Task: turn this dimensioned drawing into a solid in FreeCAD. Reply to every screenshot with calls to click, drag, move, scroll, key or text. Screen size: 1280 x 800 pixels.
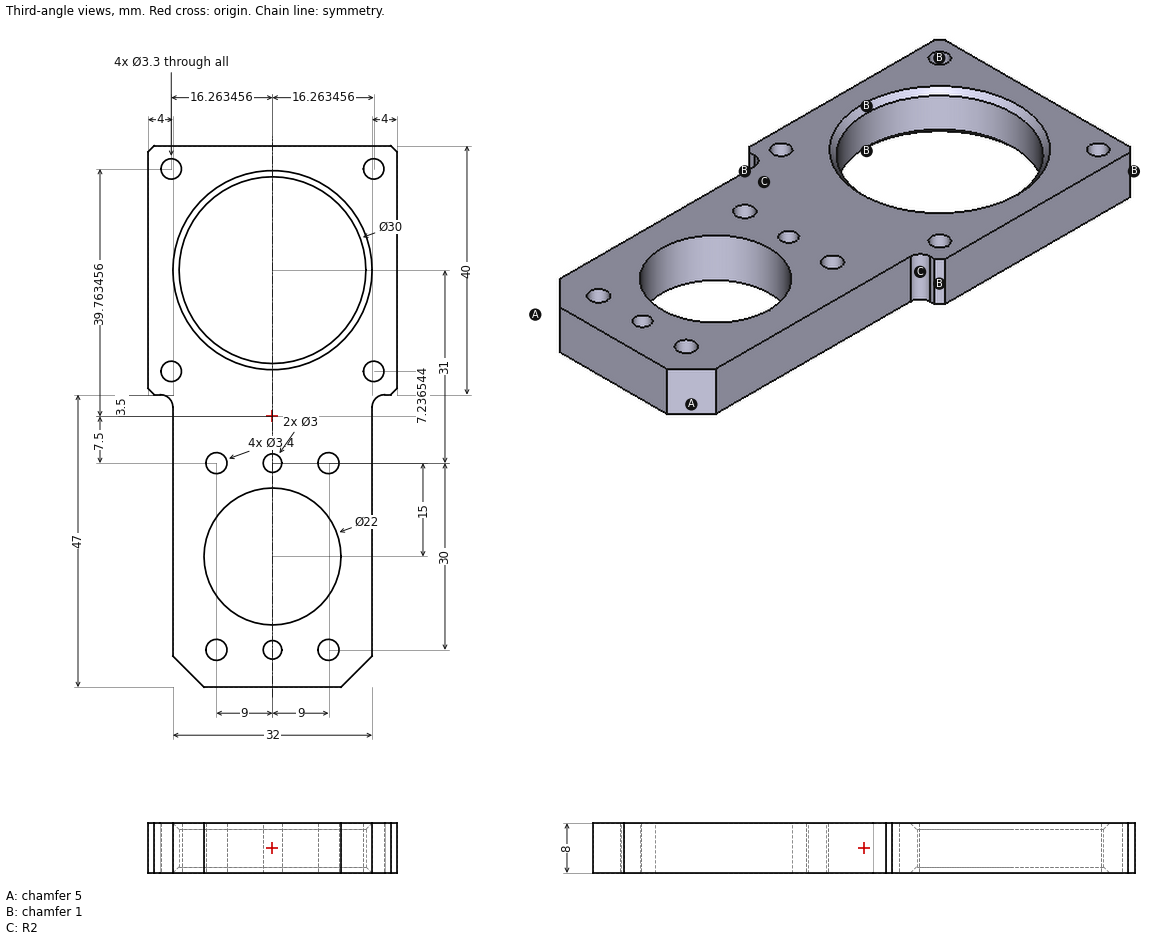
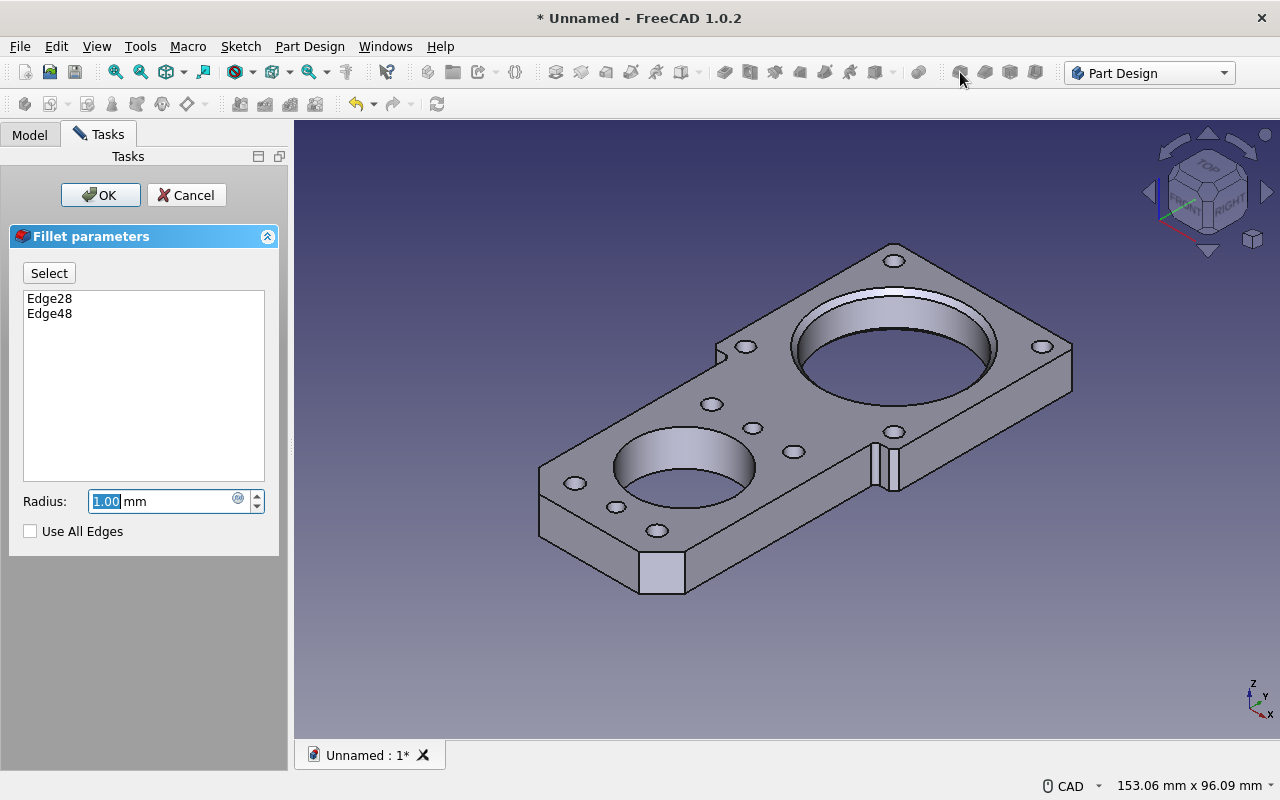
text(2)
key(Tab)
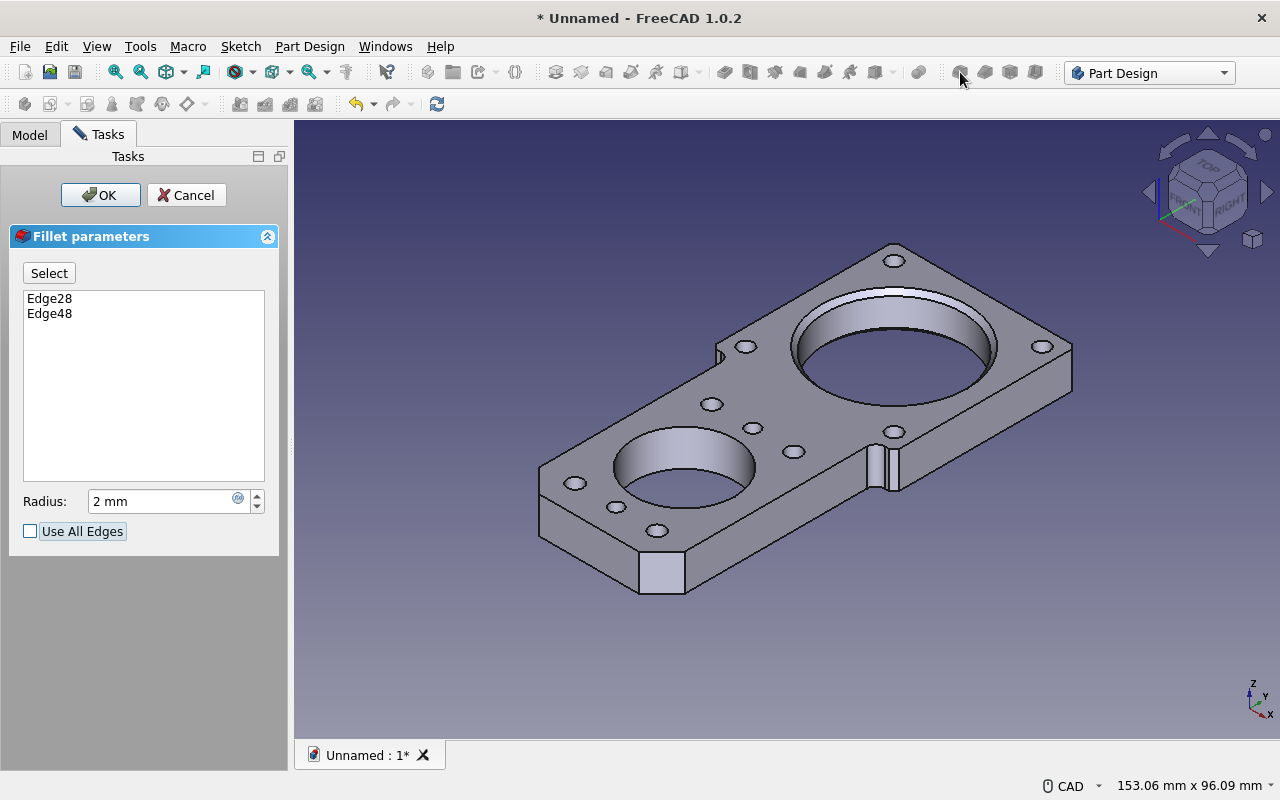
click(101, 195)